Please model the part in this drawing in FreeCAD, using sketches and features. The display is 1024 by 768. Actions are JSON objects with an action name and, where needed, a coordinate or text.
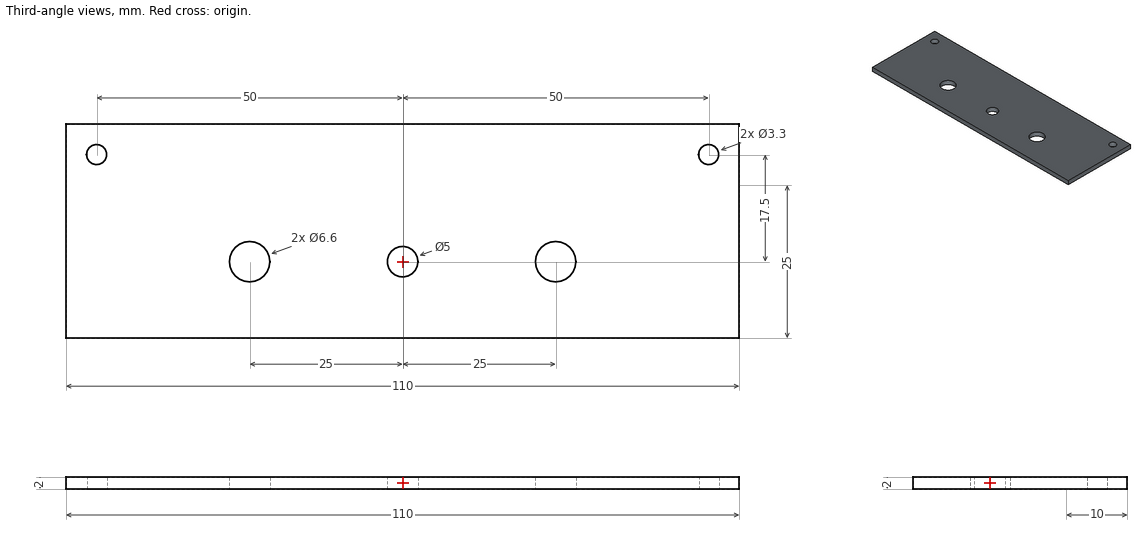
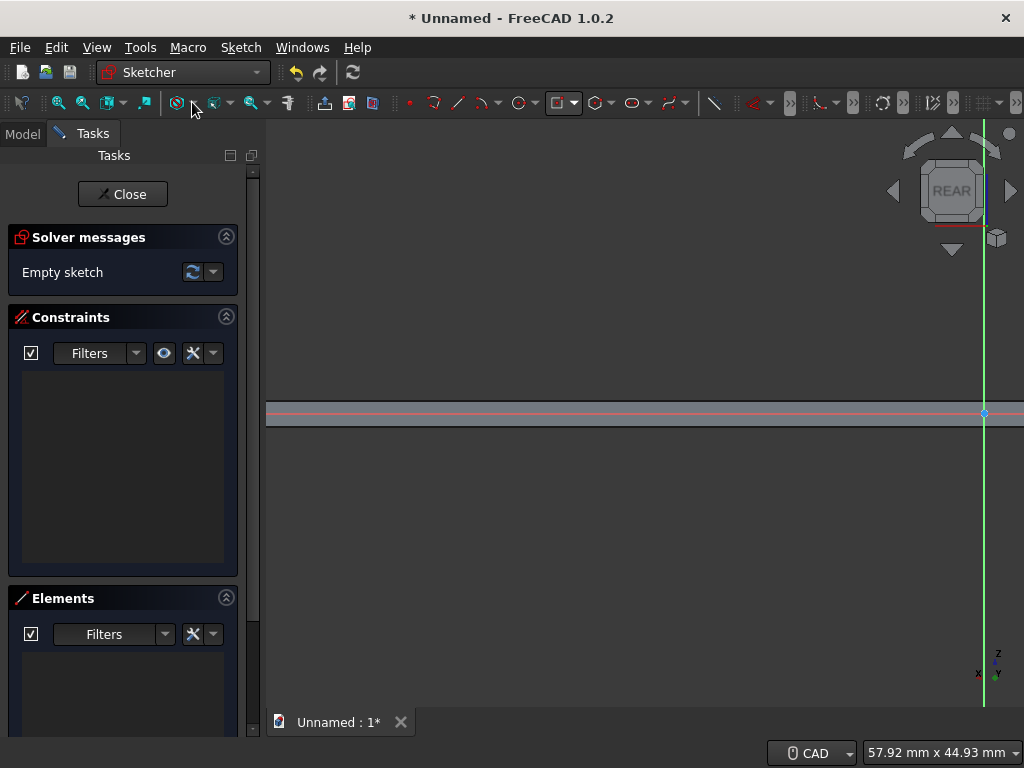
{"action": "scroll", "coordinate": [401, 413], "scroll_direction": "down", "scroll_amount": 6}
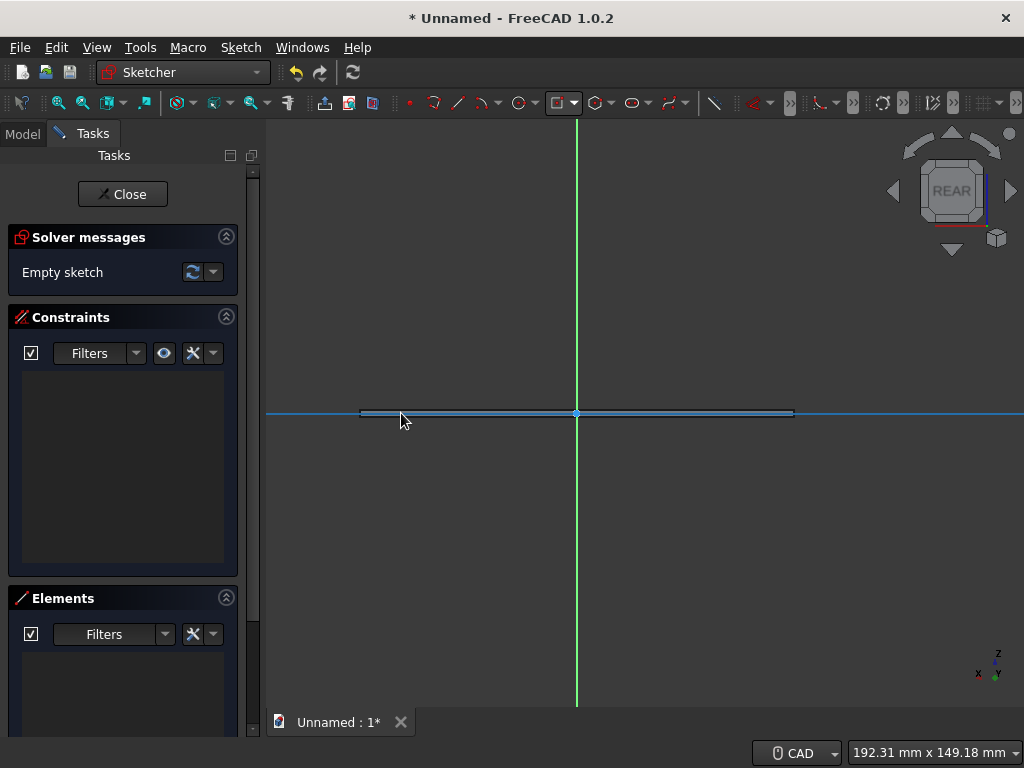
{"action": "left_click", "coordinate": [558, 104]}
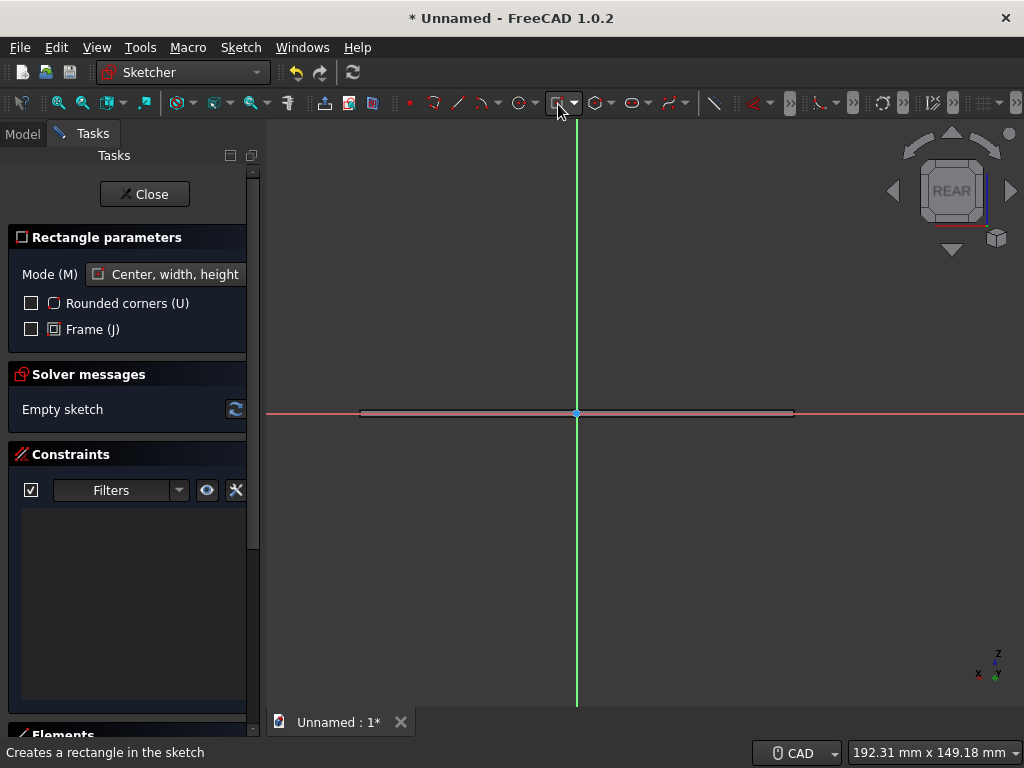
{"action": "scroll", "coordinate": [577, 414], "scroll_direction": "up", "scroll_amount": 7}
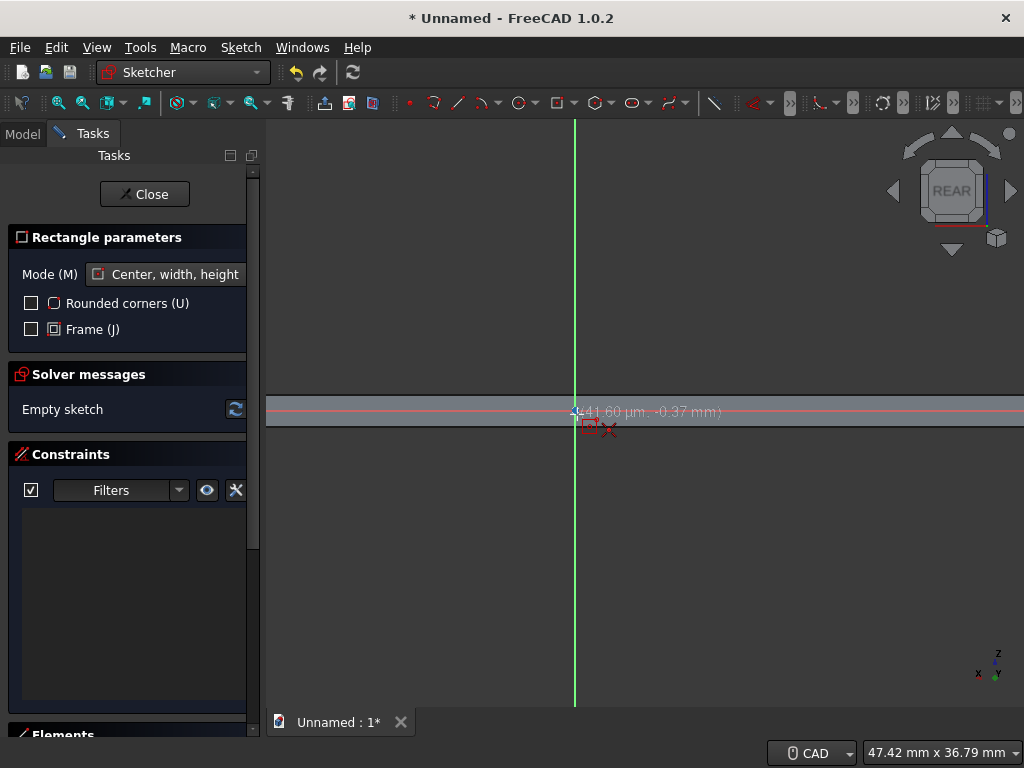
{"action": "scroll", "coordinate": [577, 414], "scroll_direction": "down", "scroll_amount": 7}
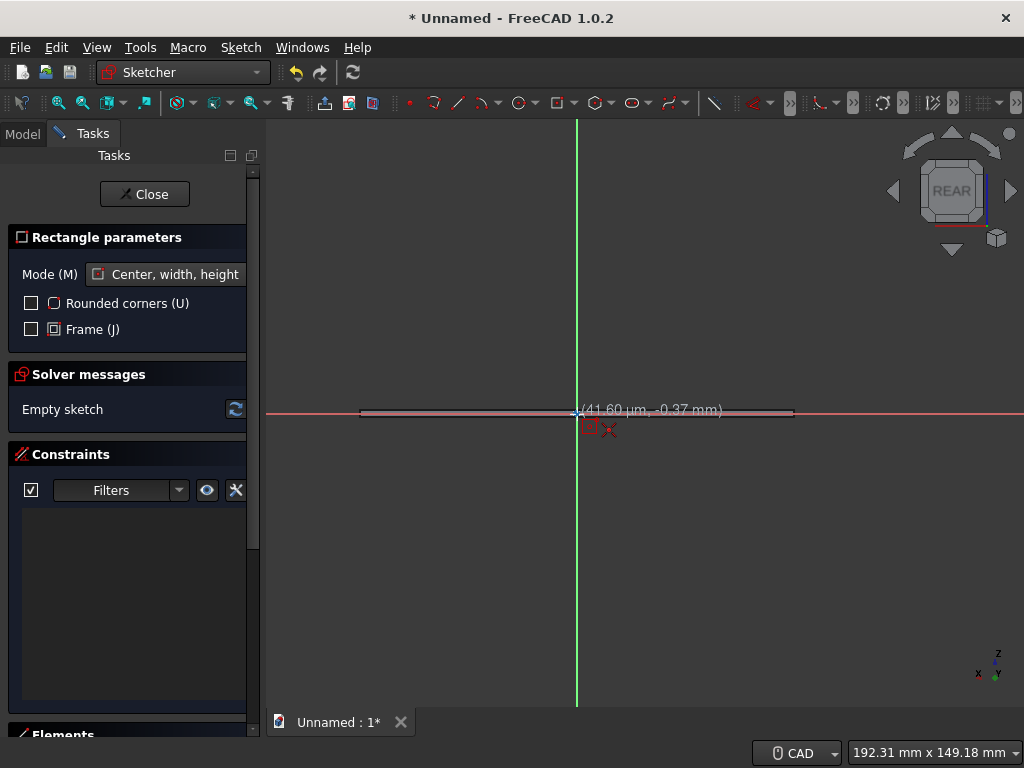
{"action": "left_click", "coordinate": [577, 414]}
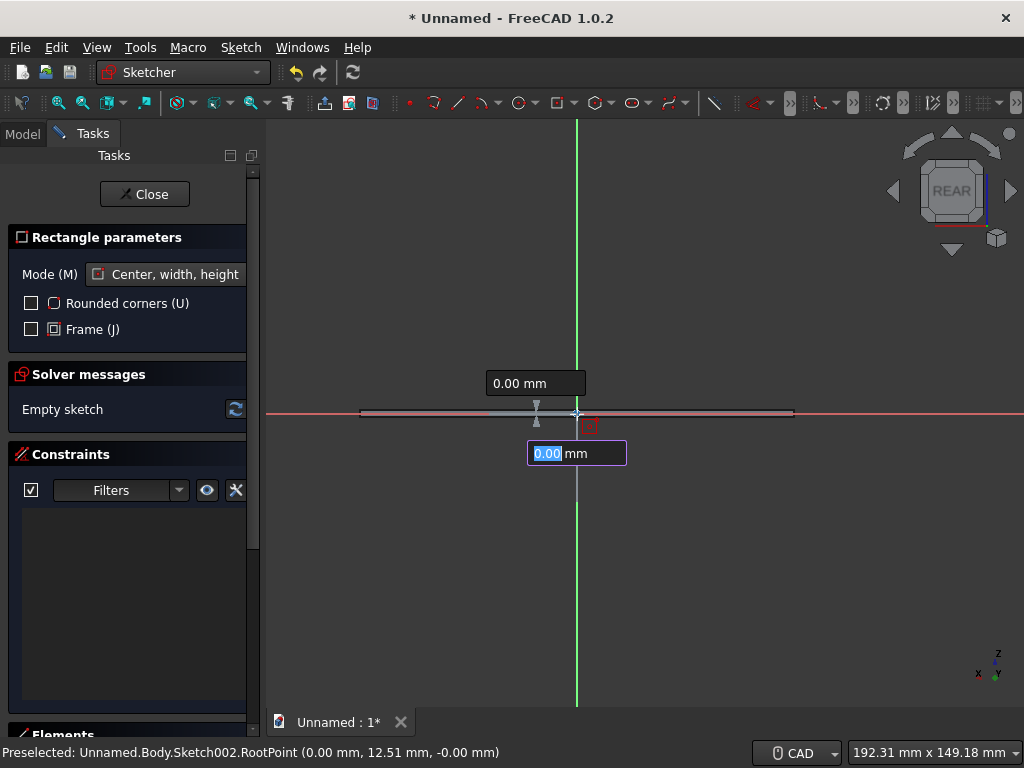
{"action": "scroll", "coordinate": [794, 410], "scroll_direction": "up", "scroll_amount": 7}
{"action": "mouse_move", "coordinate": [790, 407]}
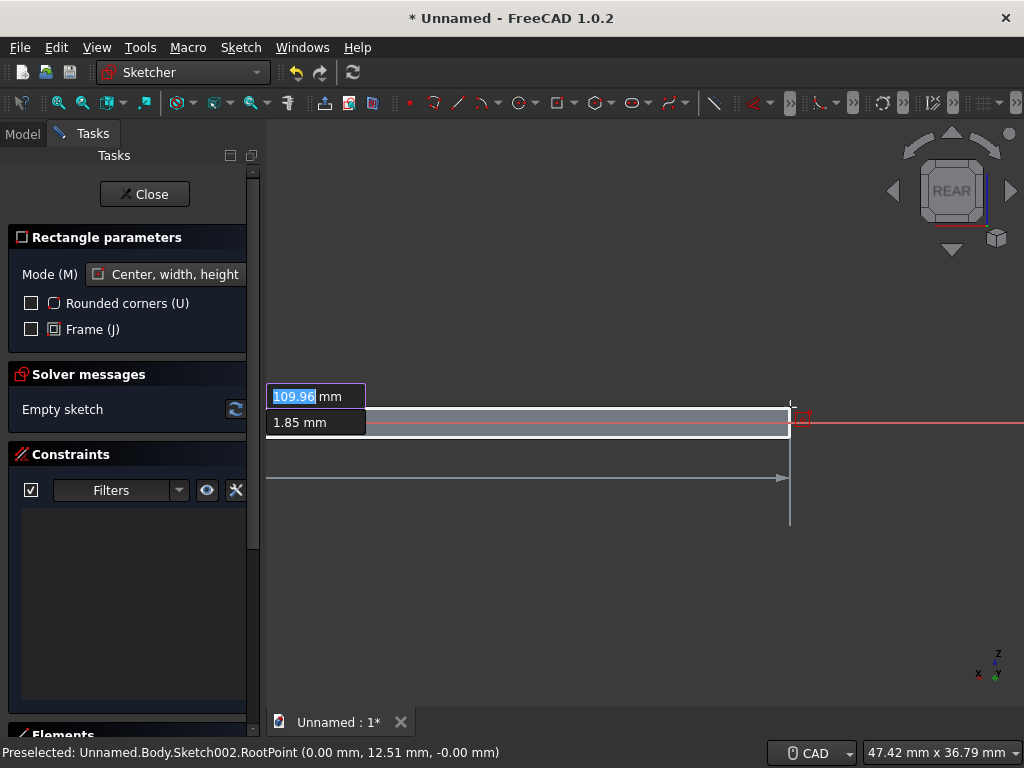
{"action": "type", "text": "110"}
{"action": "key", "text": "Tab"}
{"action": "type", "text": "2"}
{"action": "key", "text": "Return"}
{"action": "key", "text": "Escape"}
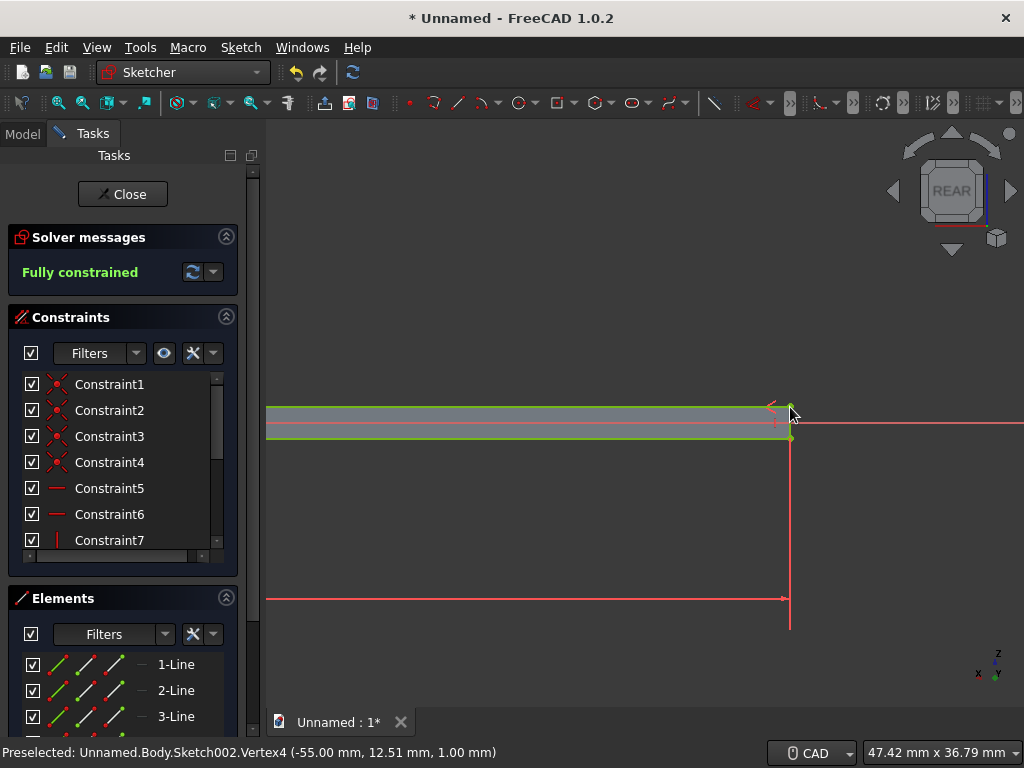
{"action": "left_click", "coordinate": [123, 194]}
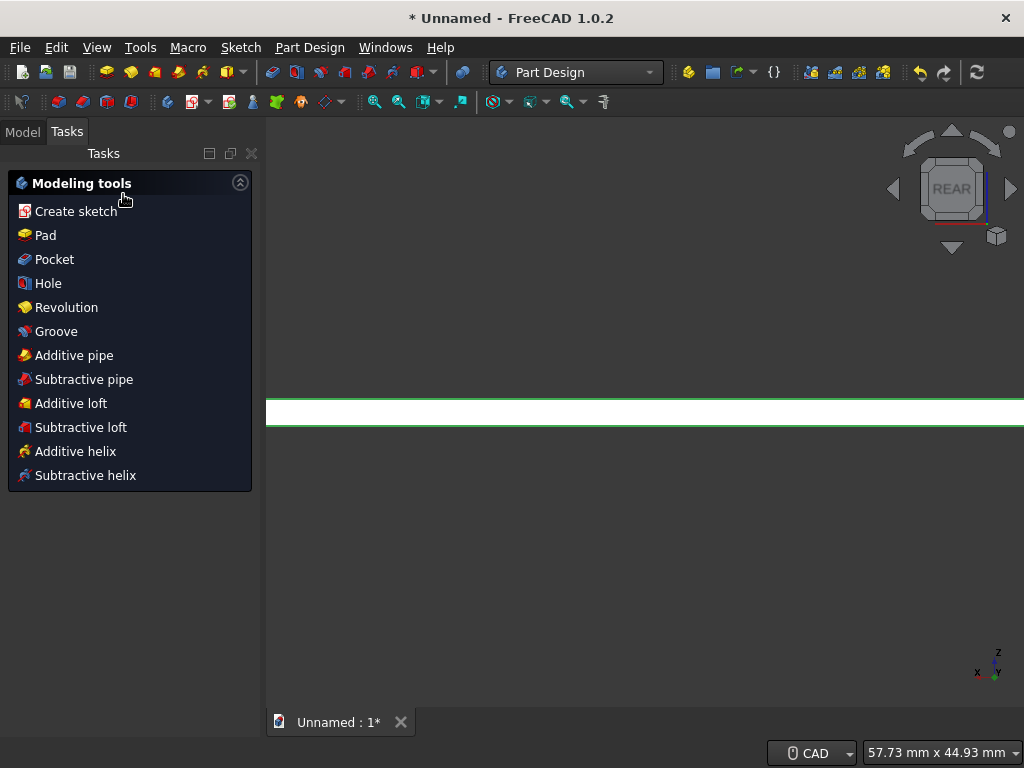
{"action": "left_click", "coordinate": [108, 72]}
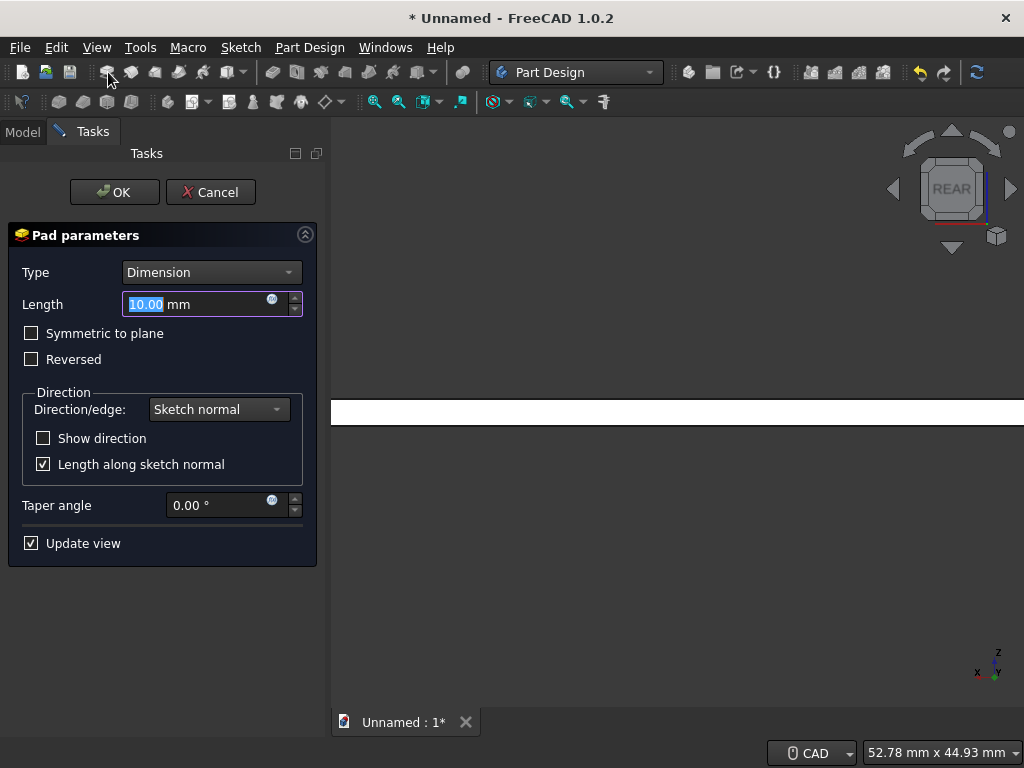
{"action": "type", "text": "10"}
{"action": "key", "text": "Tab"}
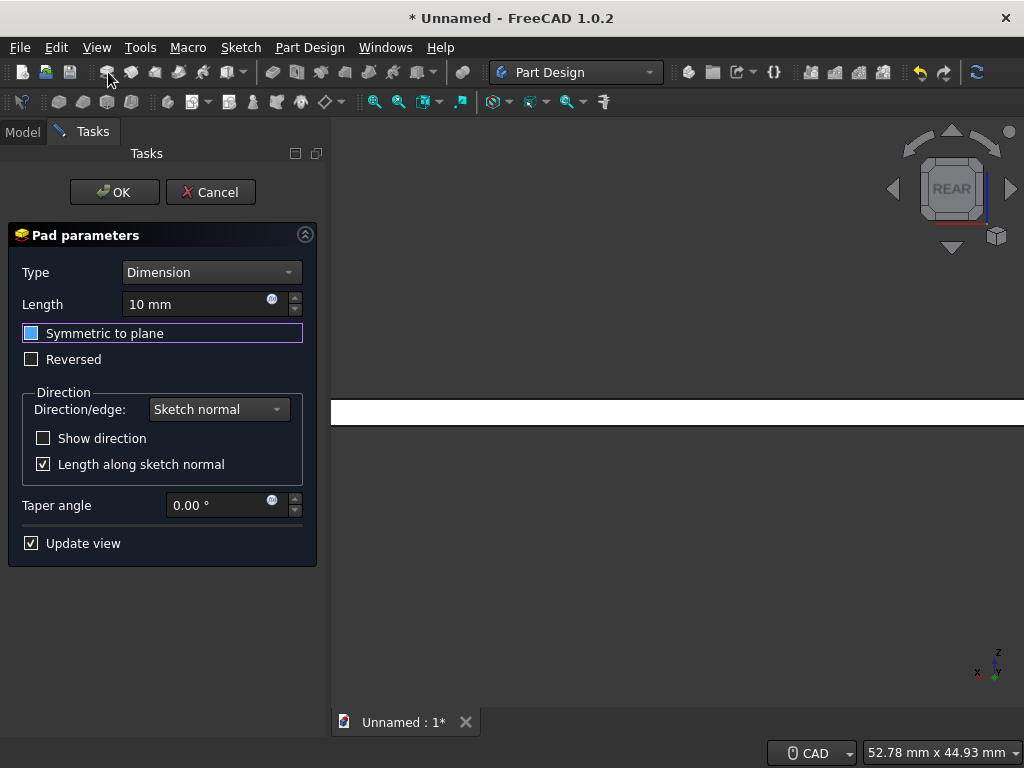
{"action": "left_click", "coordinate": [115, 192]}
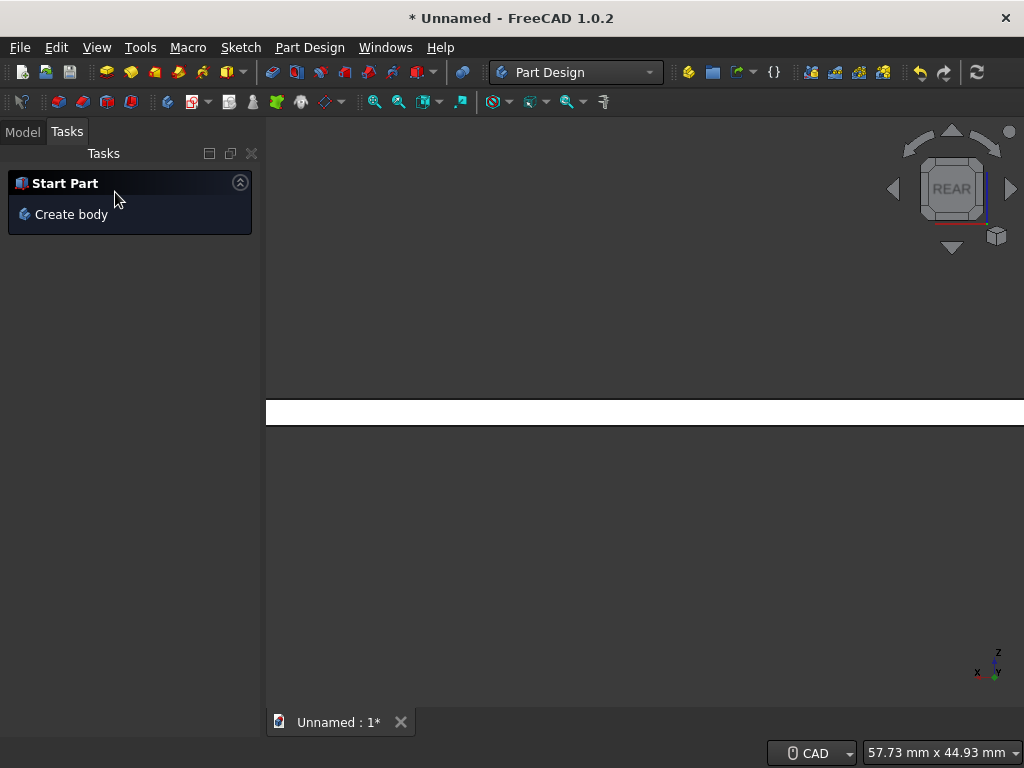
{"action": "left_click", "coordinate": [376, 102]}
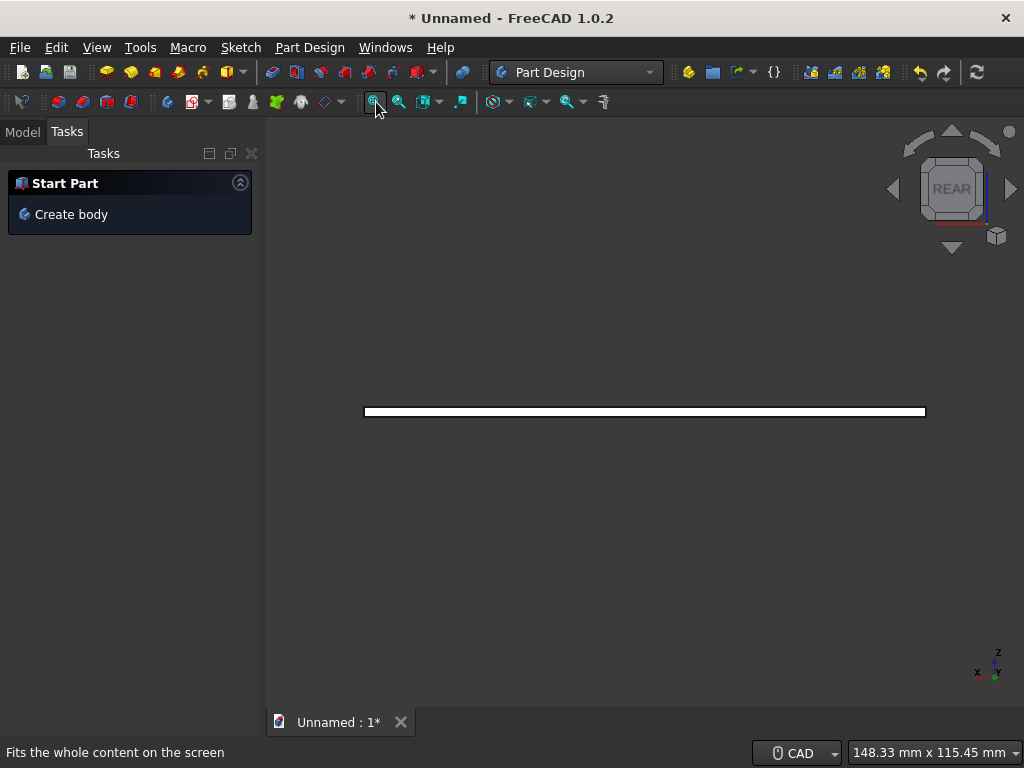
{"action": "key", "text": "5"}